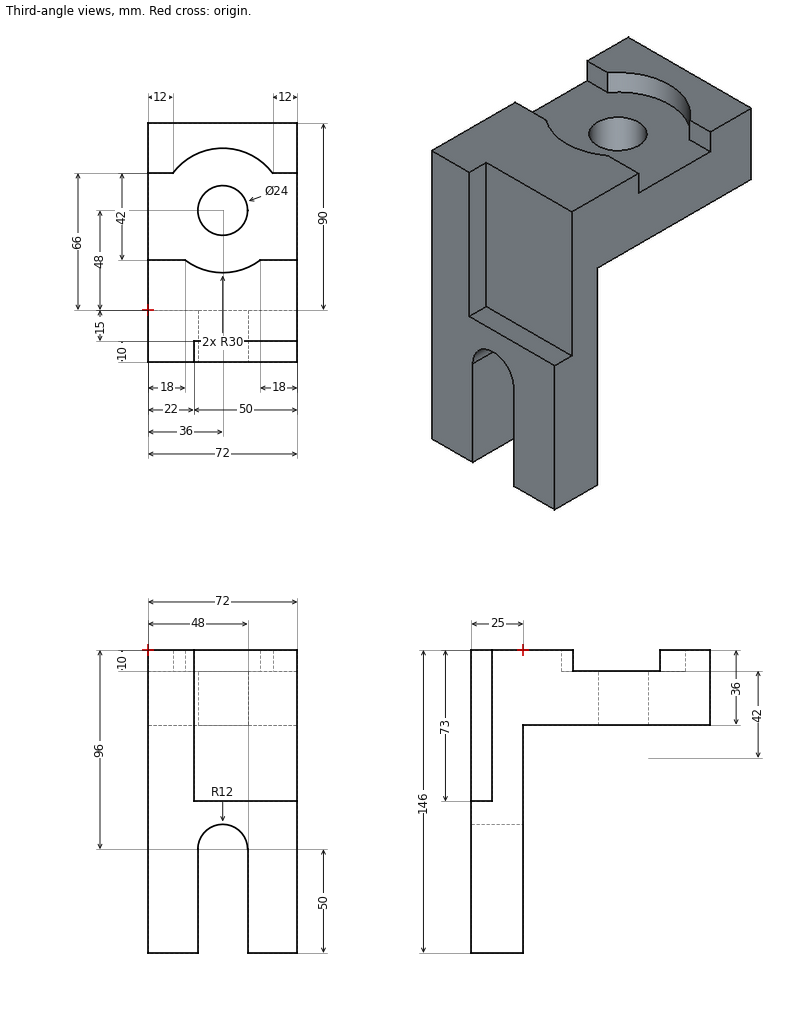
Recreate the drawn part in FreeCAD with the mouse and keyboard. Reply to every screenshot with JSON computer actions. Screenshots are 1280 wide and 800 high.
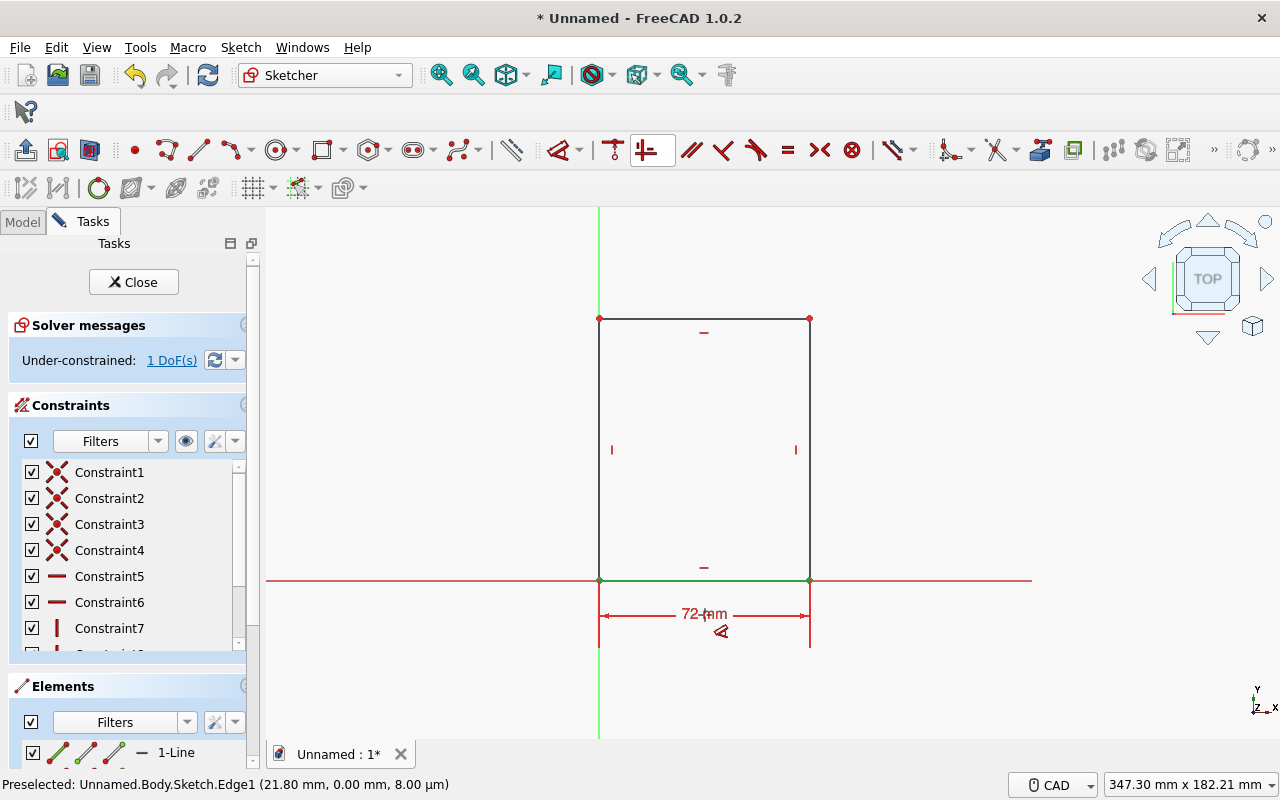
{"action": "left_click", "coordinate": [810, 502]}
{"action": "left_click", "coordinate": [844, 450]}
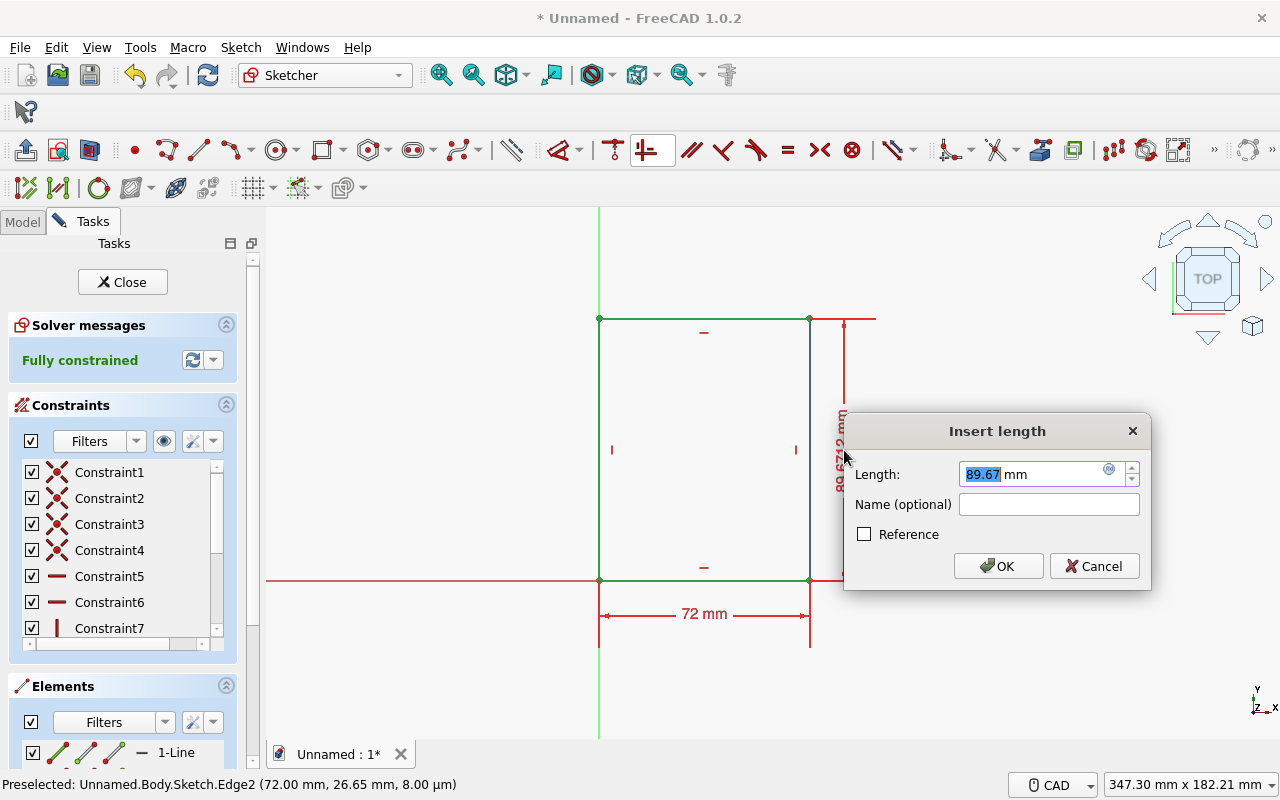
{"action": "type", "text": "90"}
{"action": "key", "text": "Return"}
{"action": "key", "text": "Escape"}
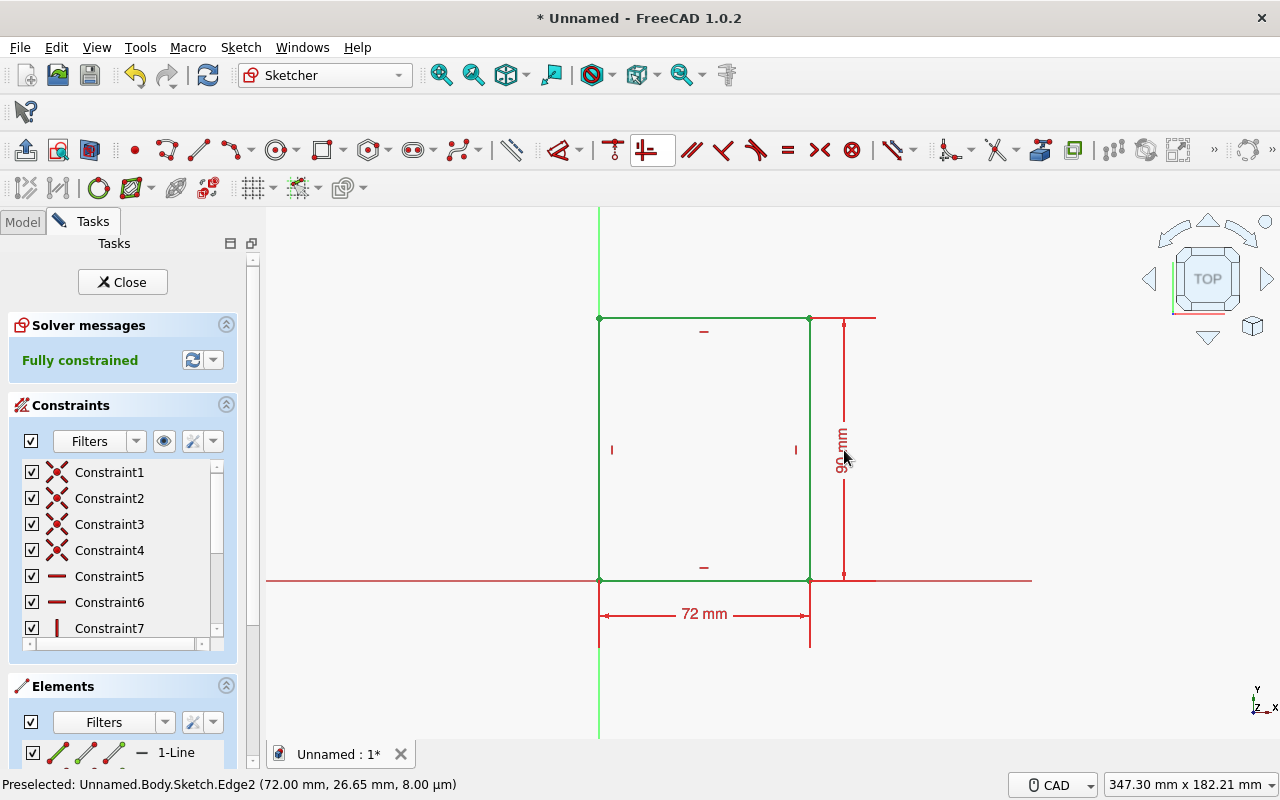
{"action": "left_click", "coordinate": [123, 282]}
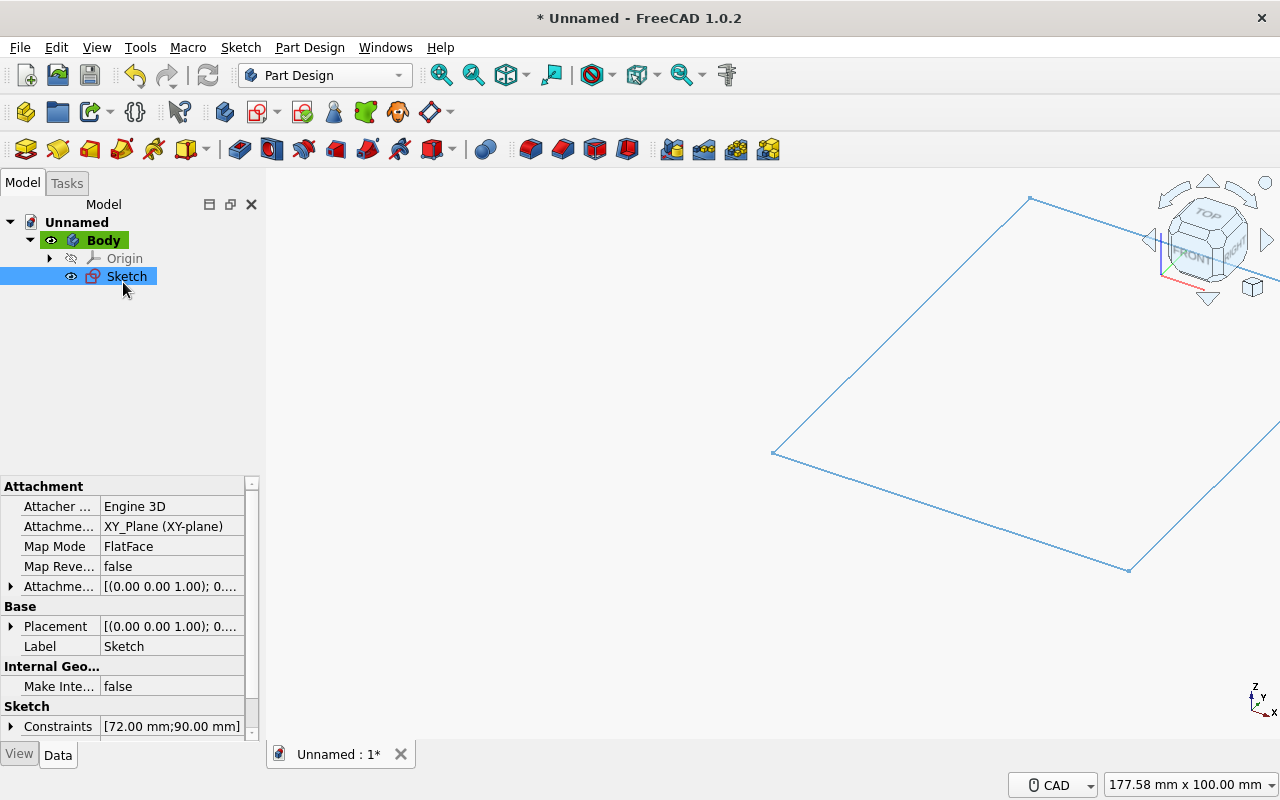
{"action": "left_click", "coordinate": [26, 150]}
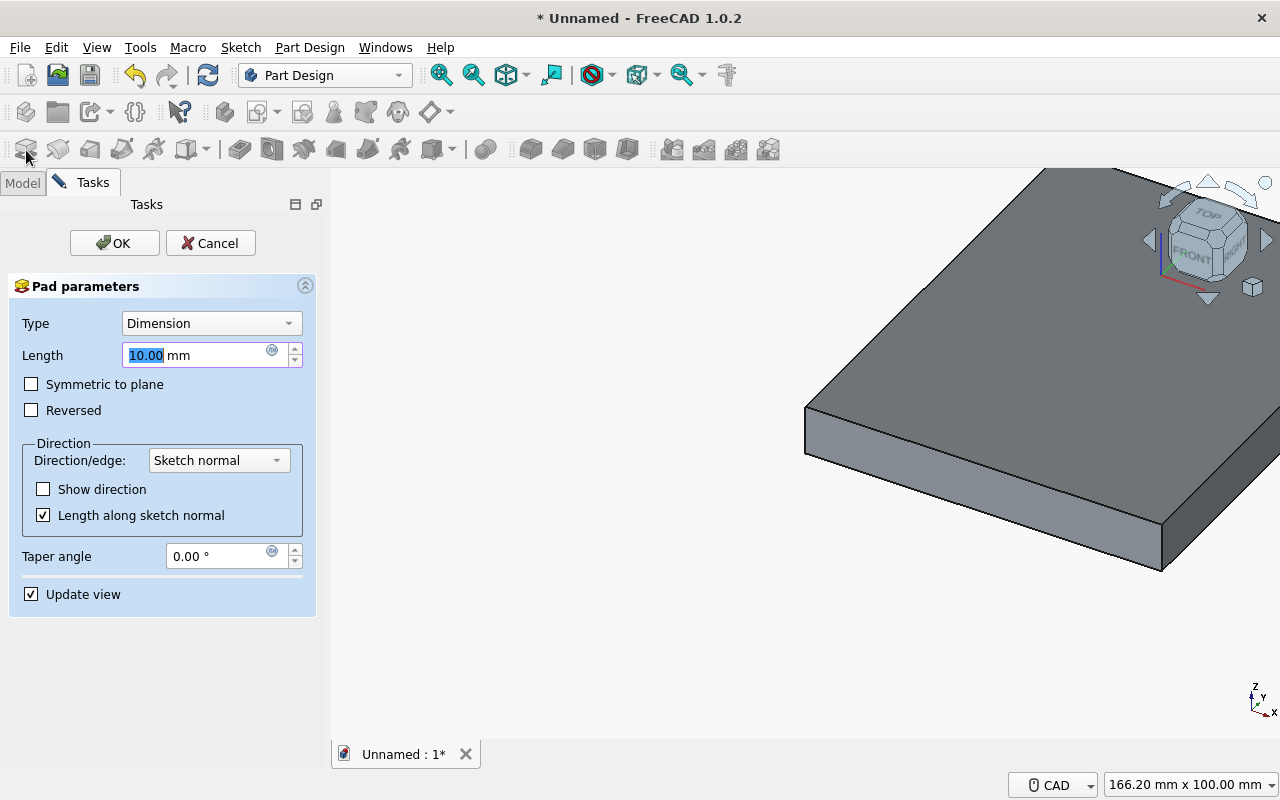
{"action": "type", "text": "36"}
{"action": "key", "text": "Tab"}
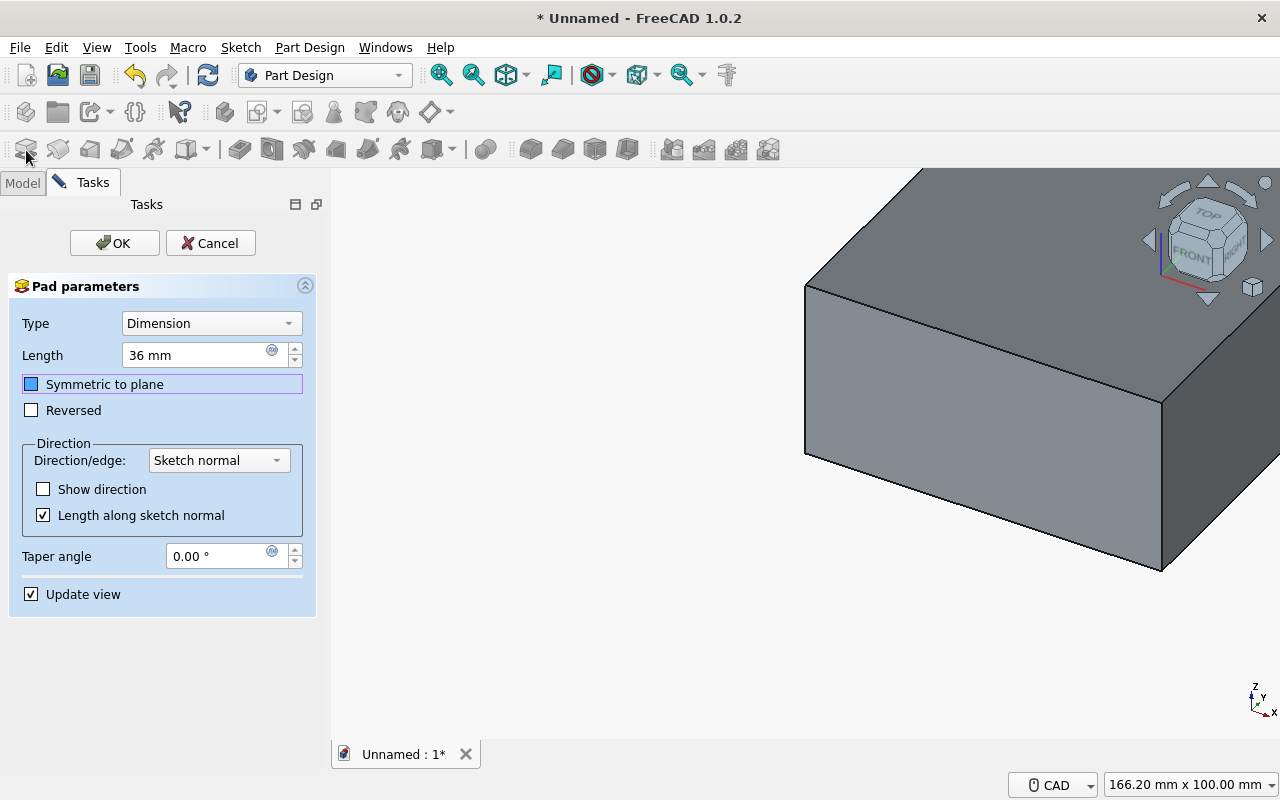
{"action": "left_click", "coordinate": [30, 410]}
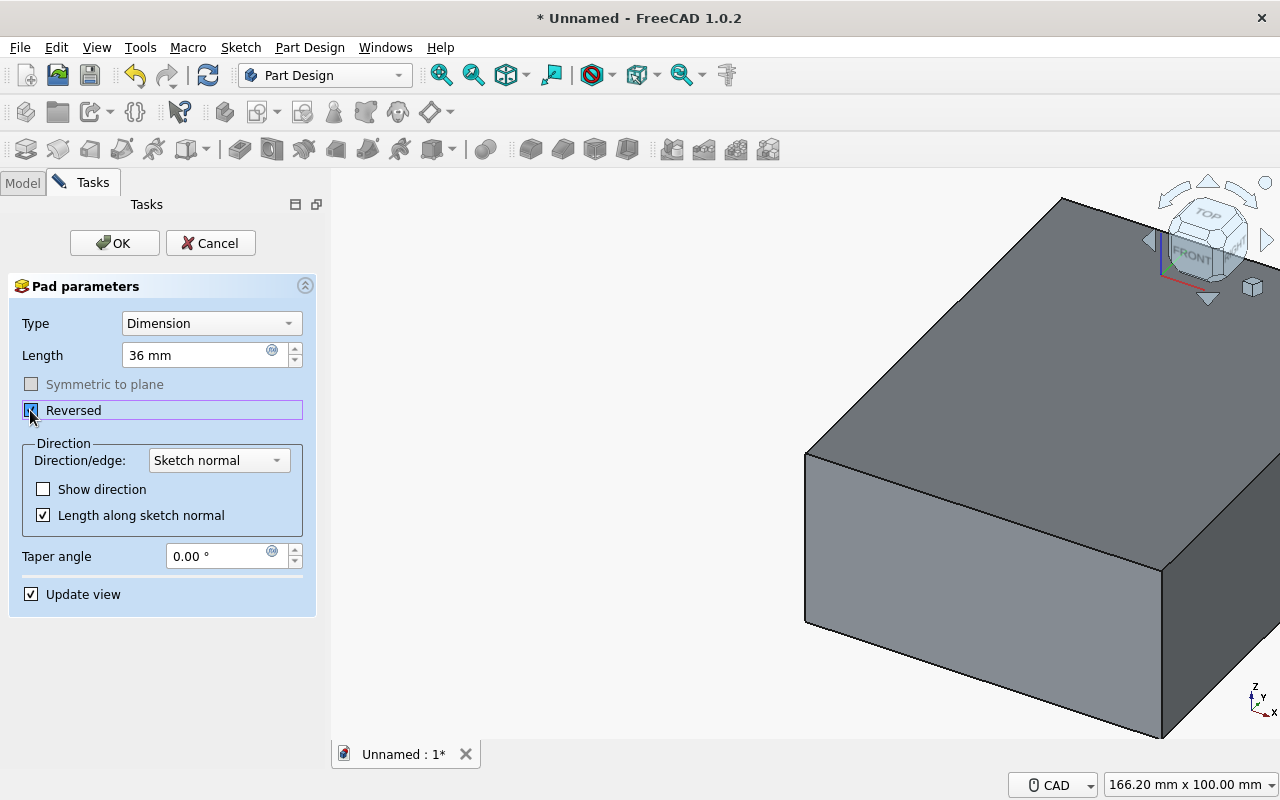
{"action": "left_click", "coordinate": [115, 243]}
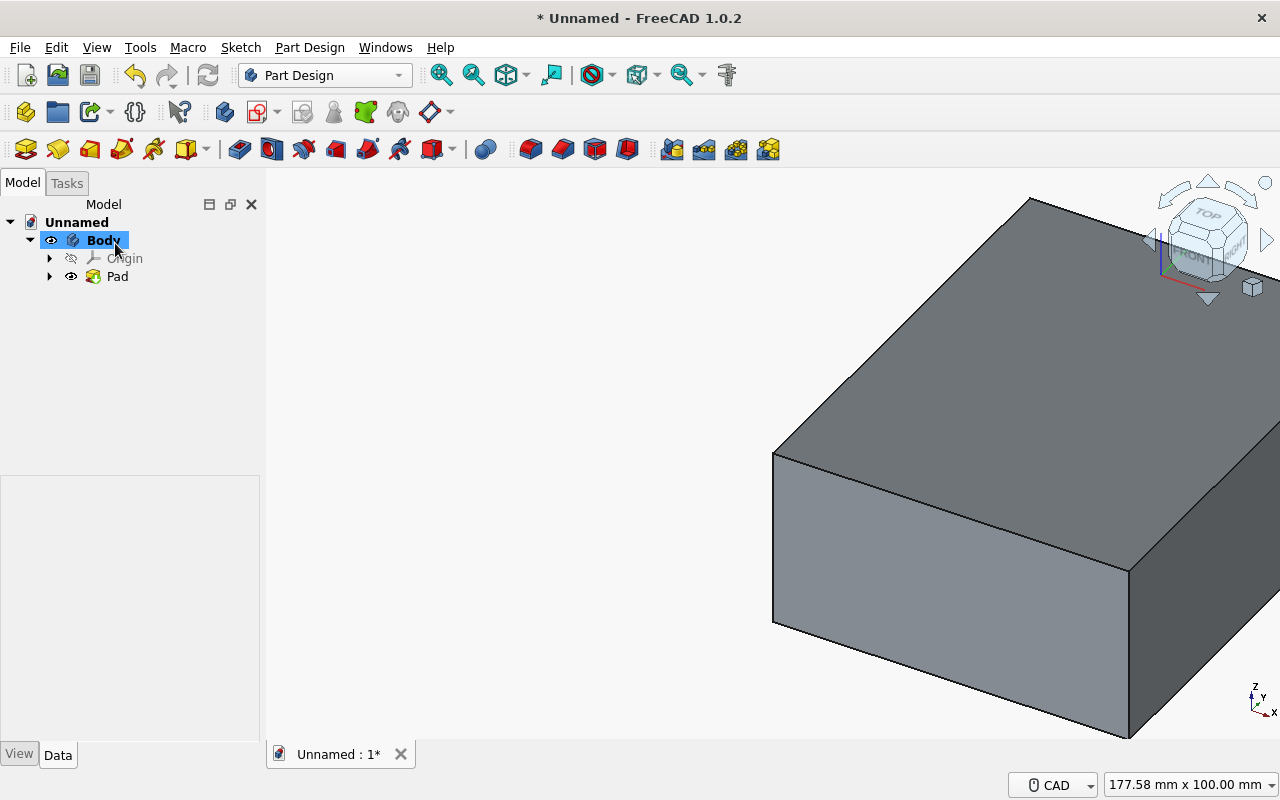
{"action": "left_click", "coordinate": [442, 76]}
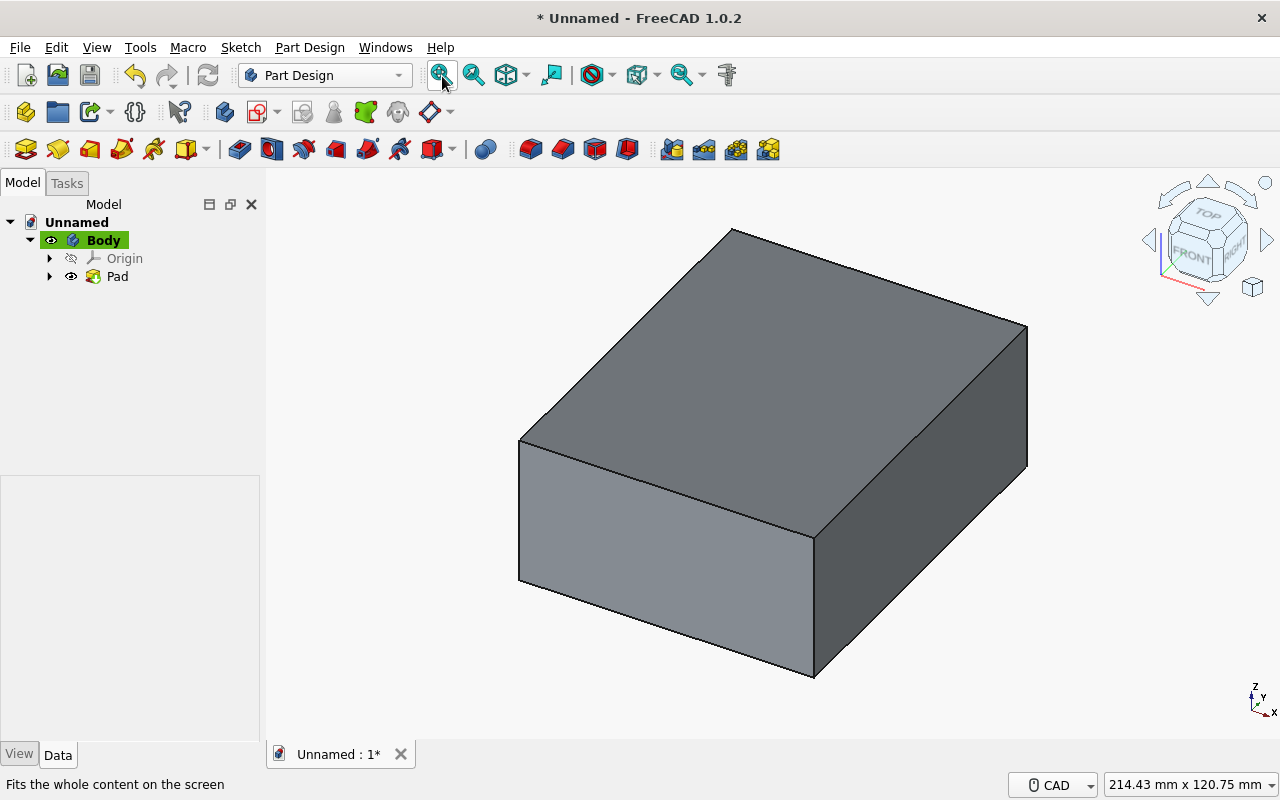
{"action": "left_click", "coordinate": [773, 383]}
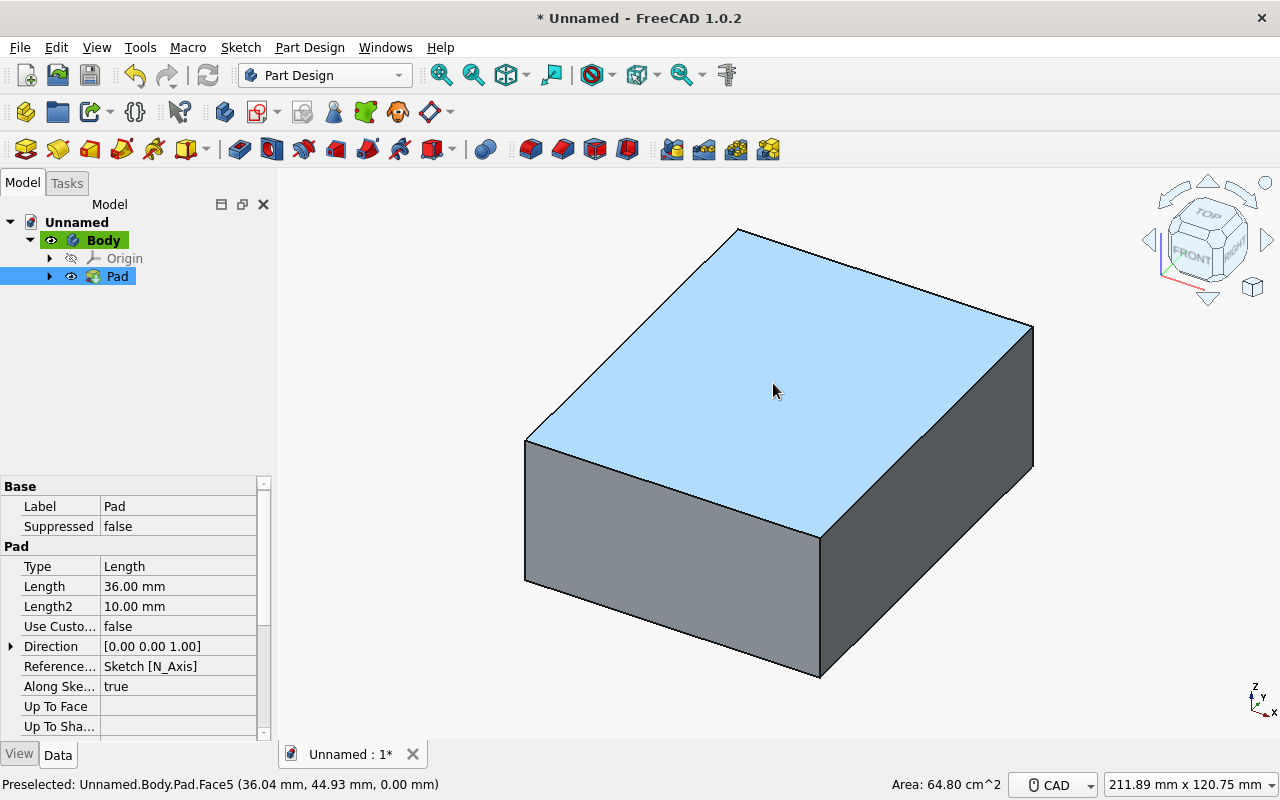
{"action": "left_click", "coordinate": [258, 112]}